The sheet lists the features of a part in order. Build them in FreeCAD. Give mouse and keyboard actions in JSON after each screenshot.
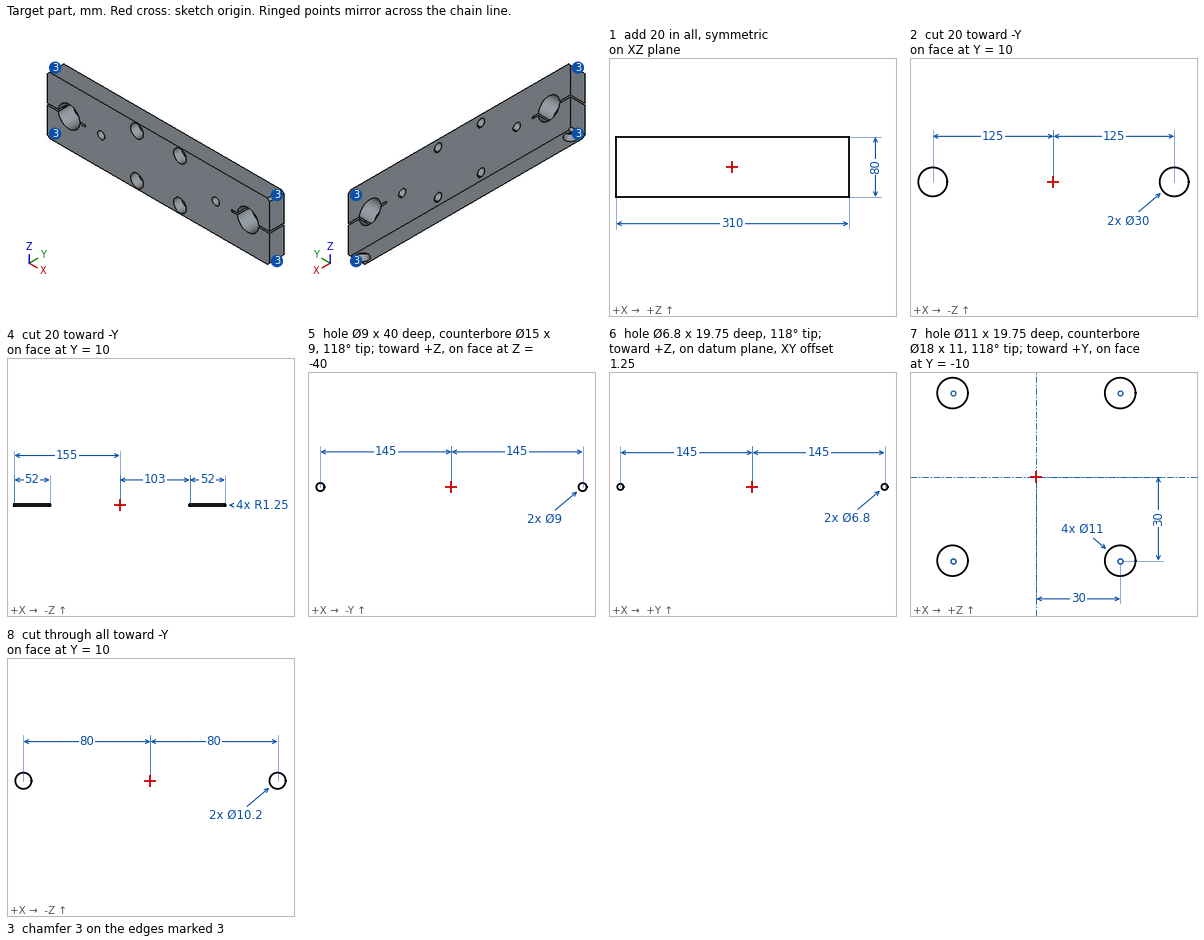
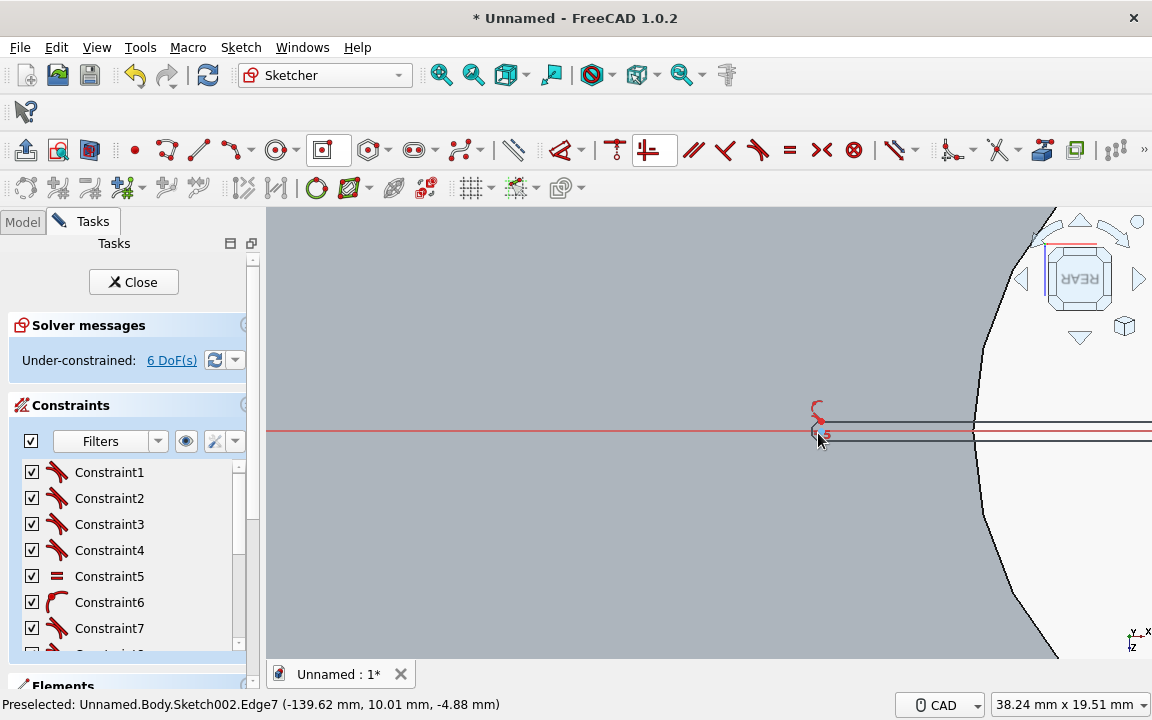
{"action": "scroll", "coordinate": [812, 431], "scroll_direction": "up", "scroll_amount": 4}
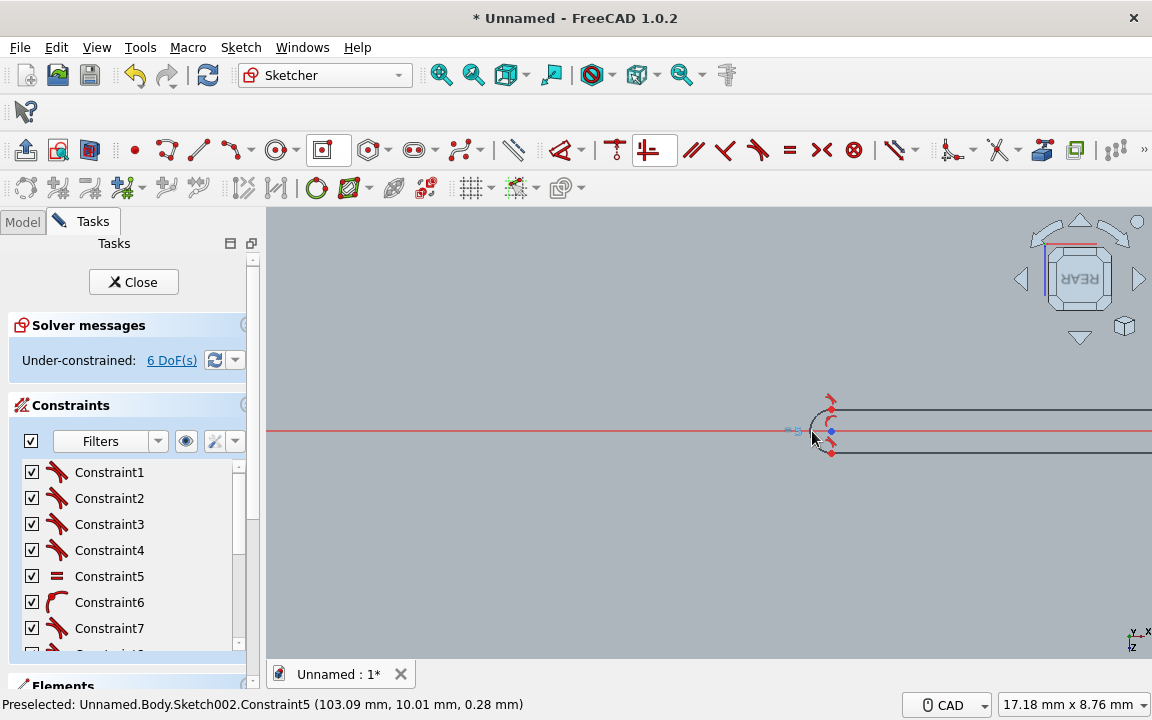
{"action": "left_click", "coordinate": [810, 431]}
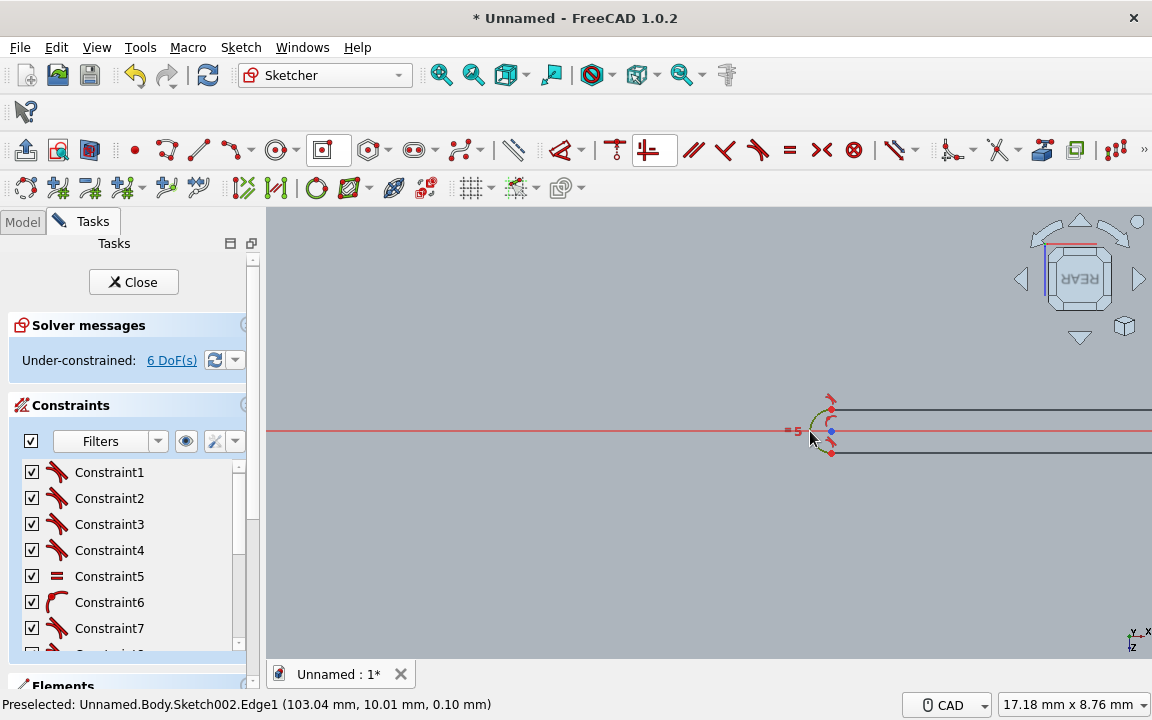
{"action": "scroll", "coordinate": [818, 433], "scroll_direction": "down", "scroll_amount": 17}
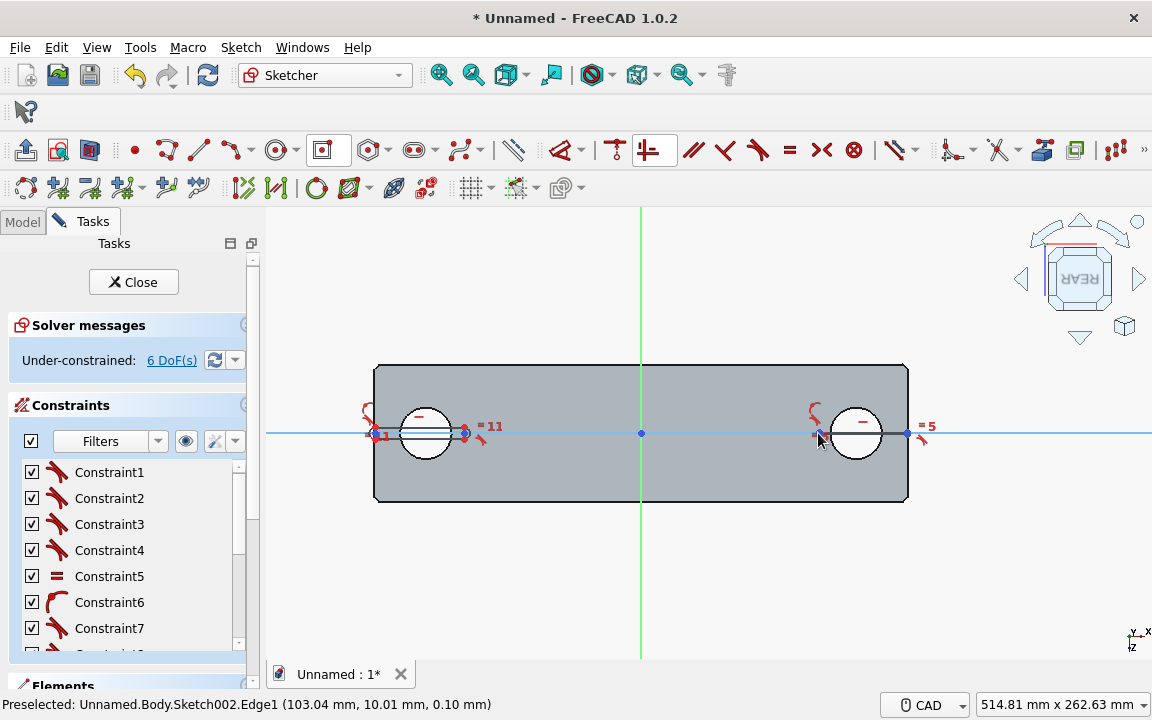
{"action": "scroll", "coordinate": [370, 430], "scroll_direction": "up", "scroll_amount": 7}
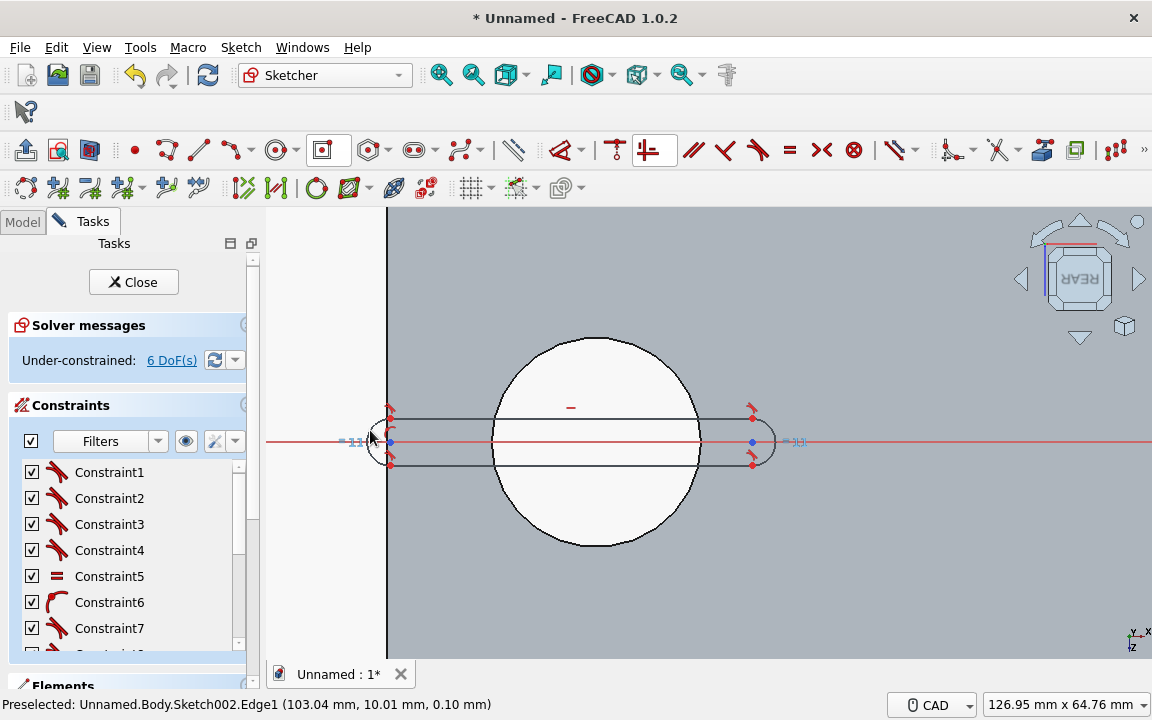
{"action": "left_click", "coordinate": [372, 429]}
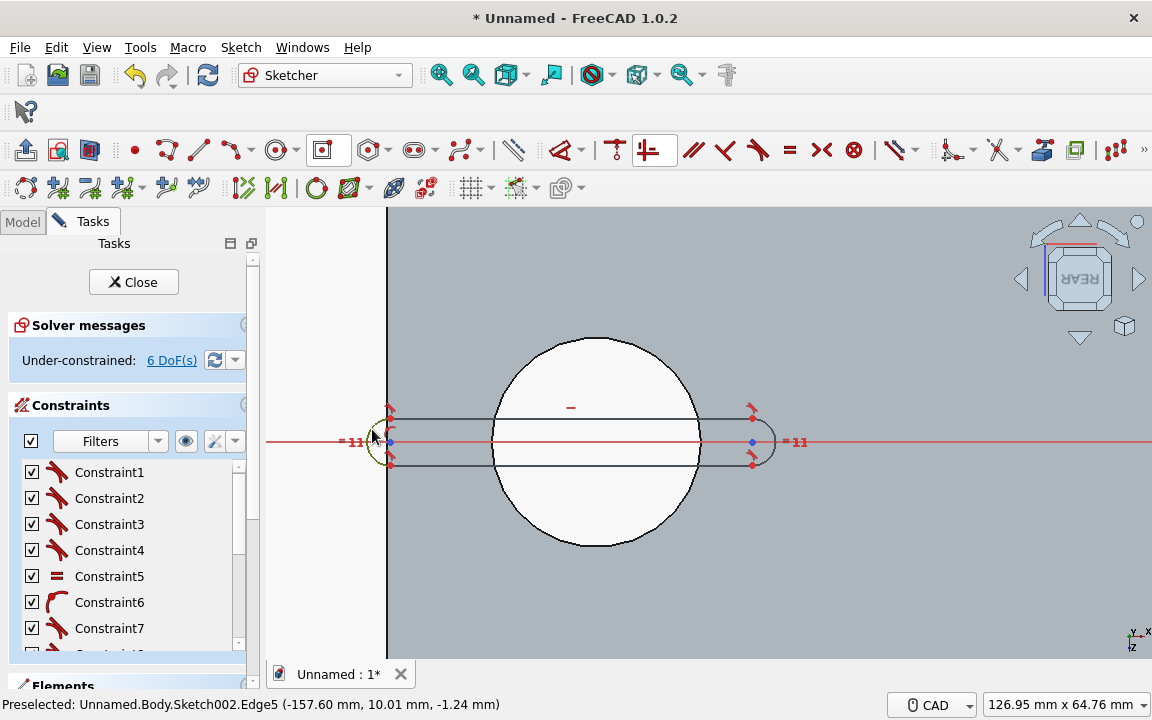
{"action": "left_click", "coordinate": [790, 150]}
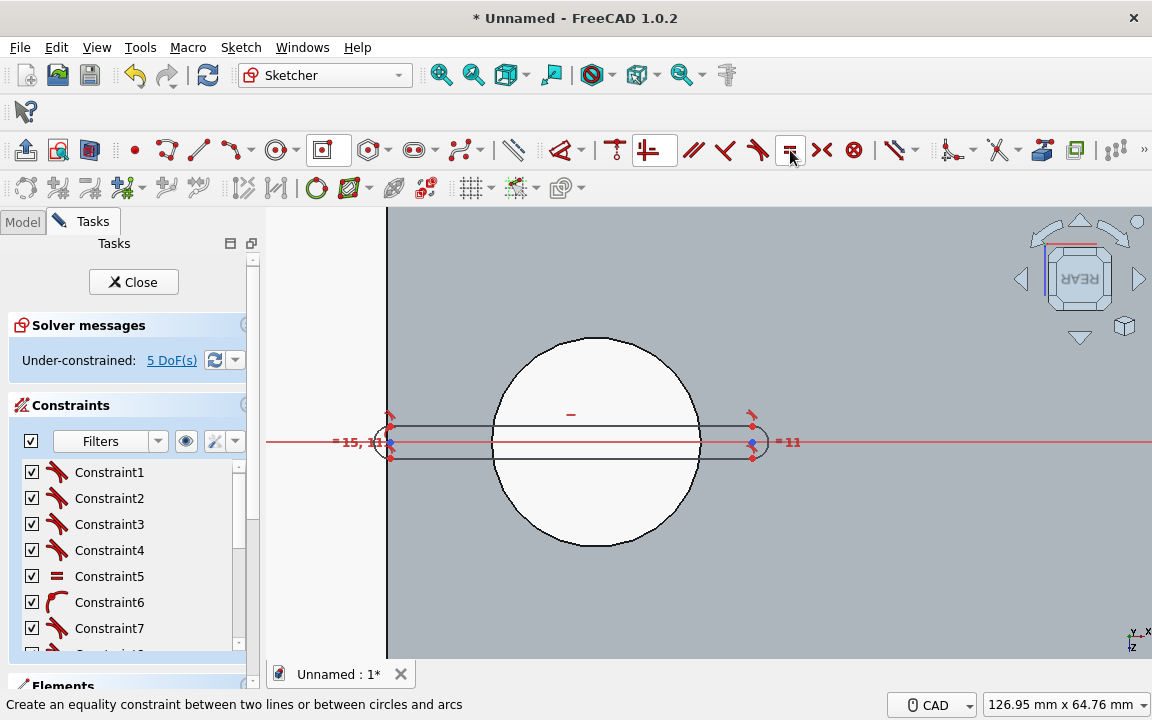
{"action": "left_click", "coordinate": [560, 150]}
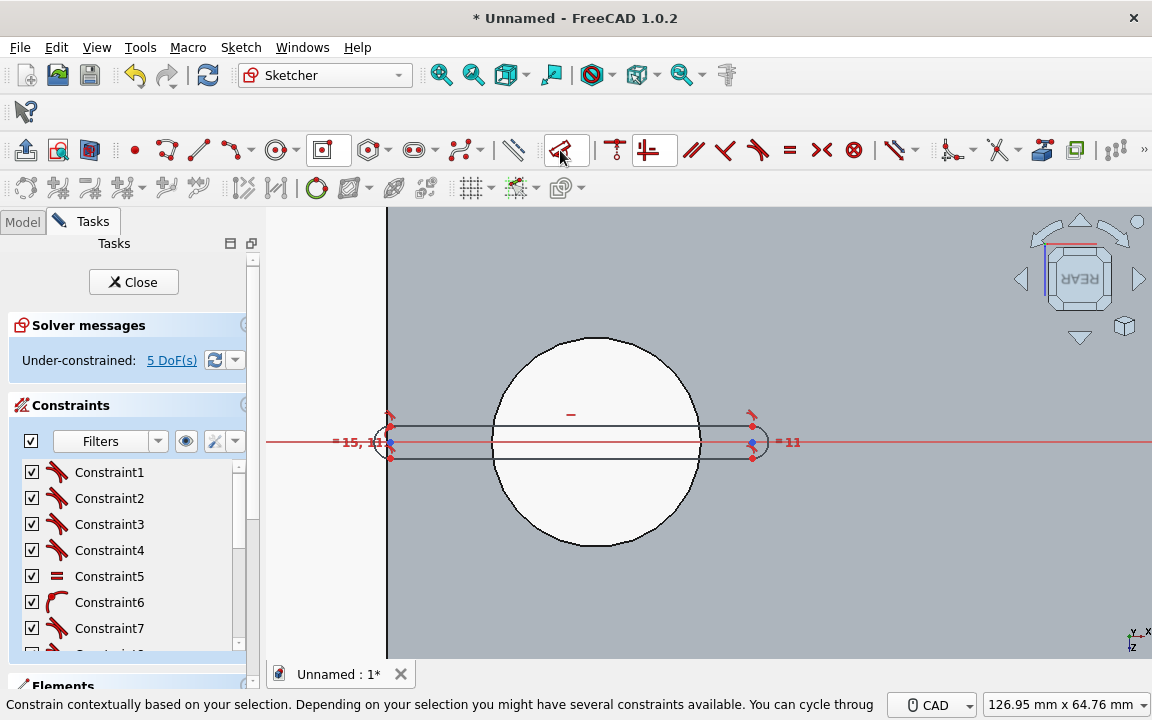
{"action": "scroll", "coordinate": [369, 430], "scroll_direction": "down", "scroll_amount": 7}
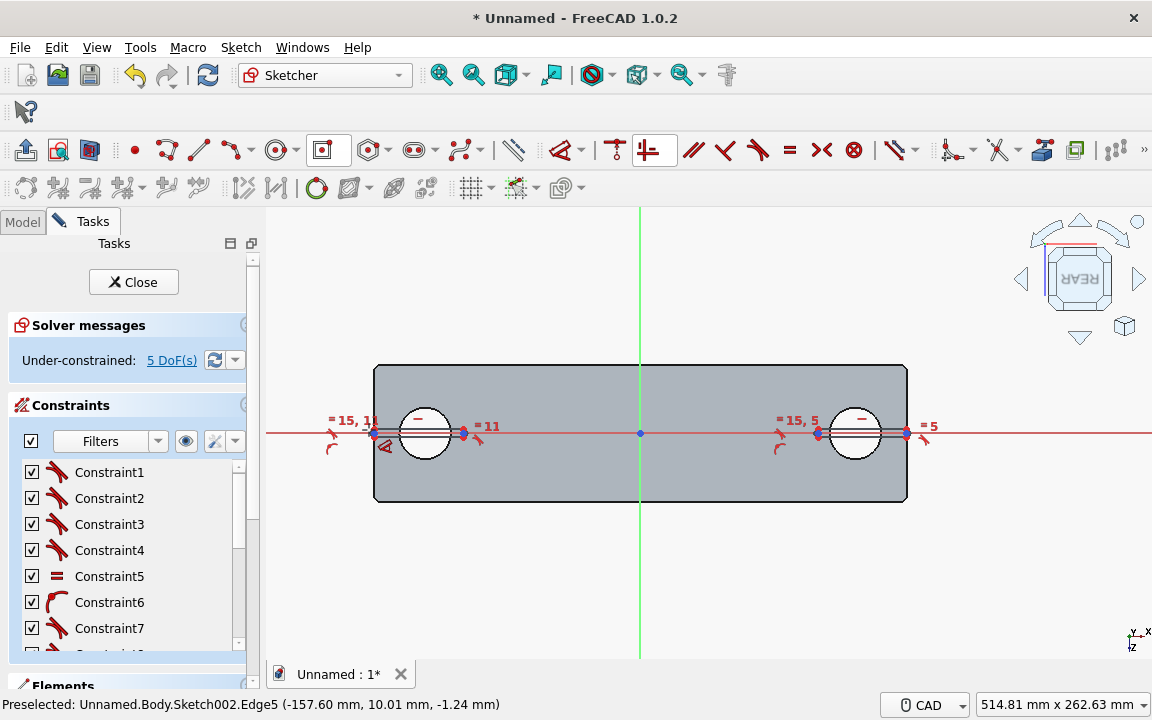
{"action": "scroll", "coordinate": [815, 431], "scroll_direction": "up", "scroll_amount": 15}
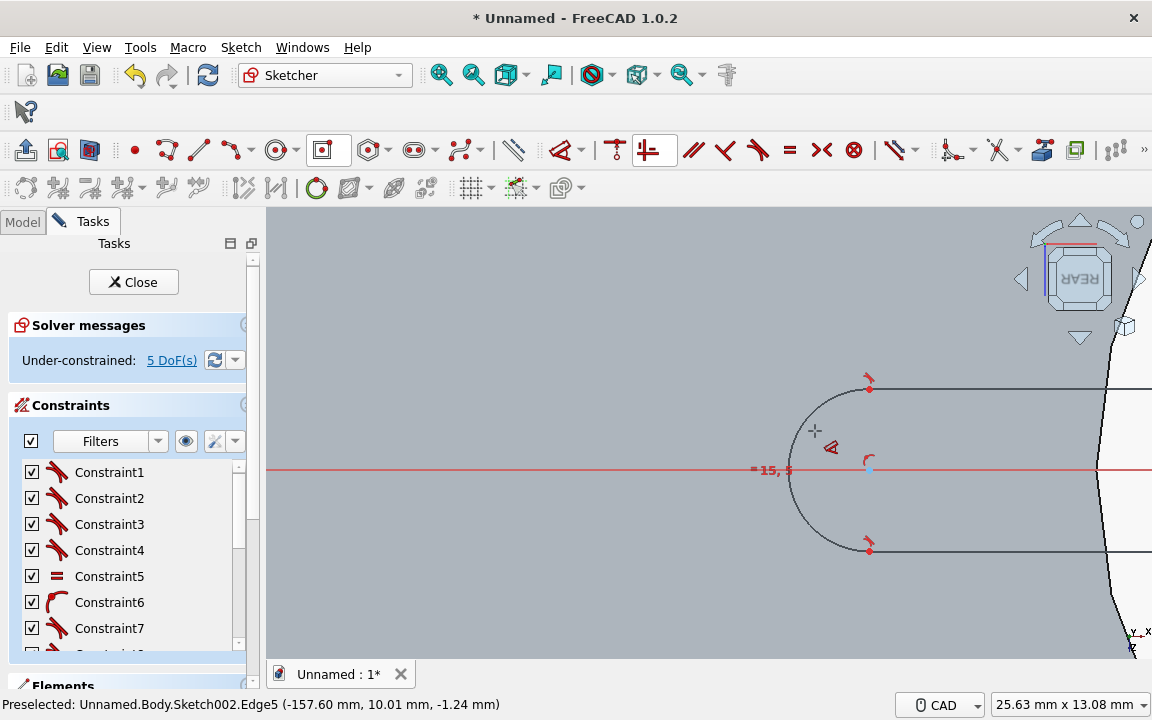
{"action": "left_click", "coordinate": [804, 423]}
{"action": "left_click", "coordinate": [778, 404]}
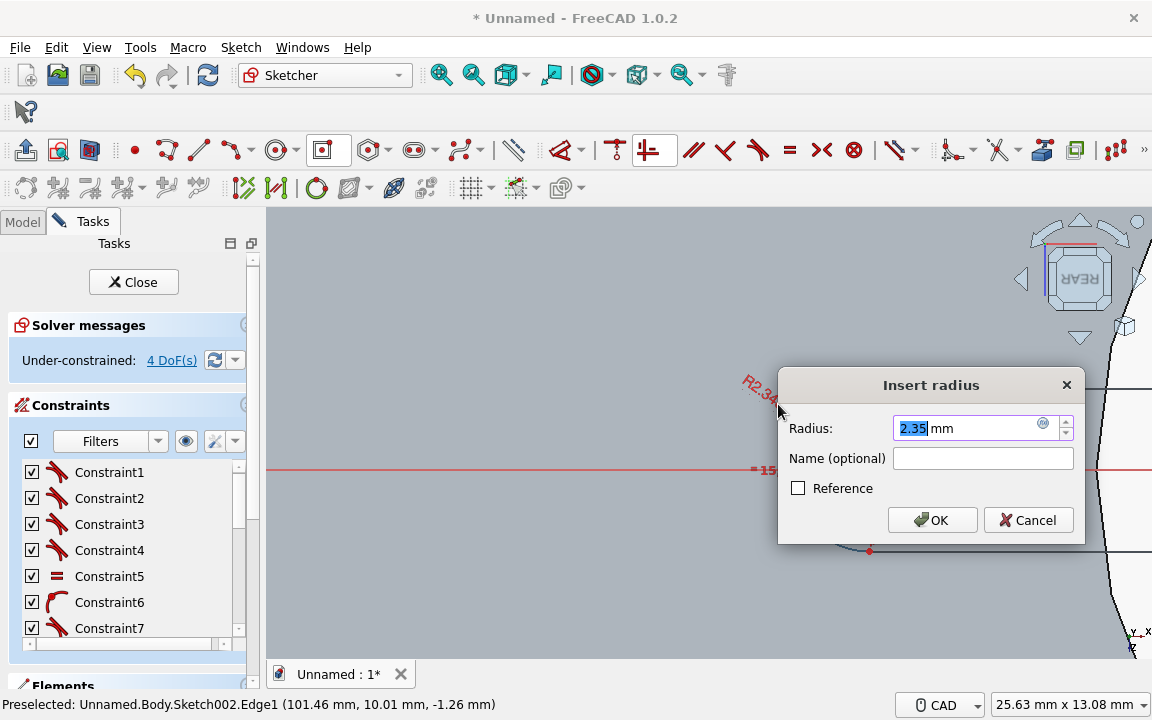
{"action": "type", "text": "1.25"}
{"action": "key", "text": "Return"}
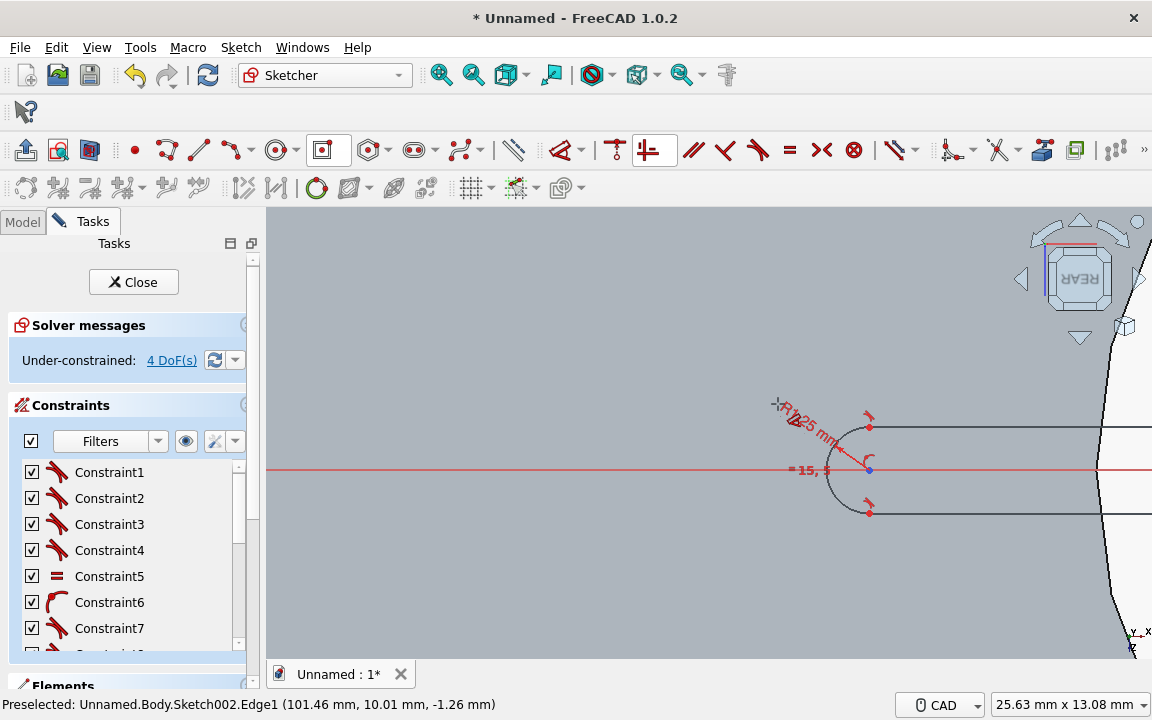
{"action": "scroll", "coordinate": [816, 431], "scroll_direction": "down", "scroll_amount": 15}